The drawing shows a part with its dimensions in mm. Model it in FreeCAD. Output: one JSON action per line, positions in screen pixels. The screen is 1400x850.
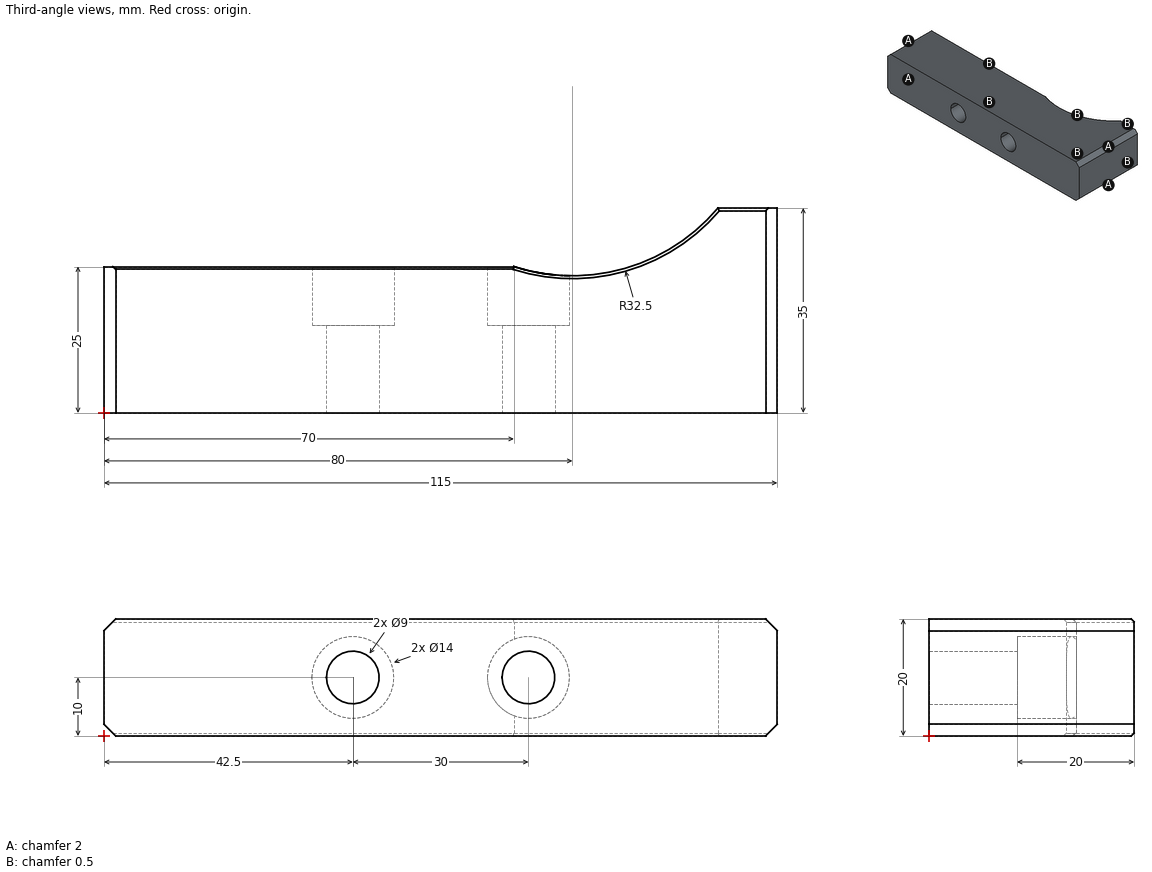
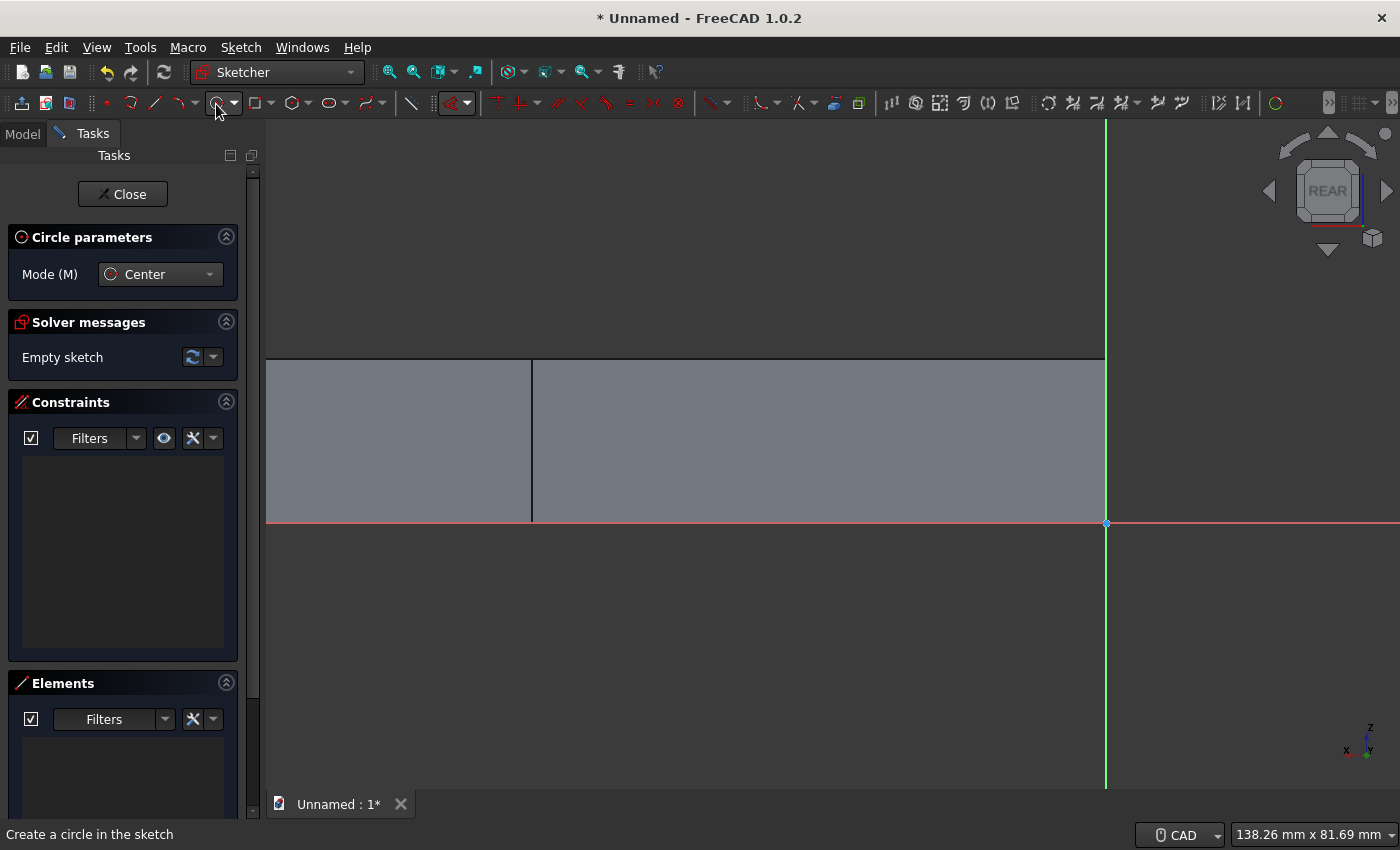
{"action": "left_click", "coordinate": [758, 441]}
{"action": "left_click", "coordinate": [798, 401]}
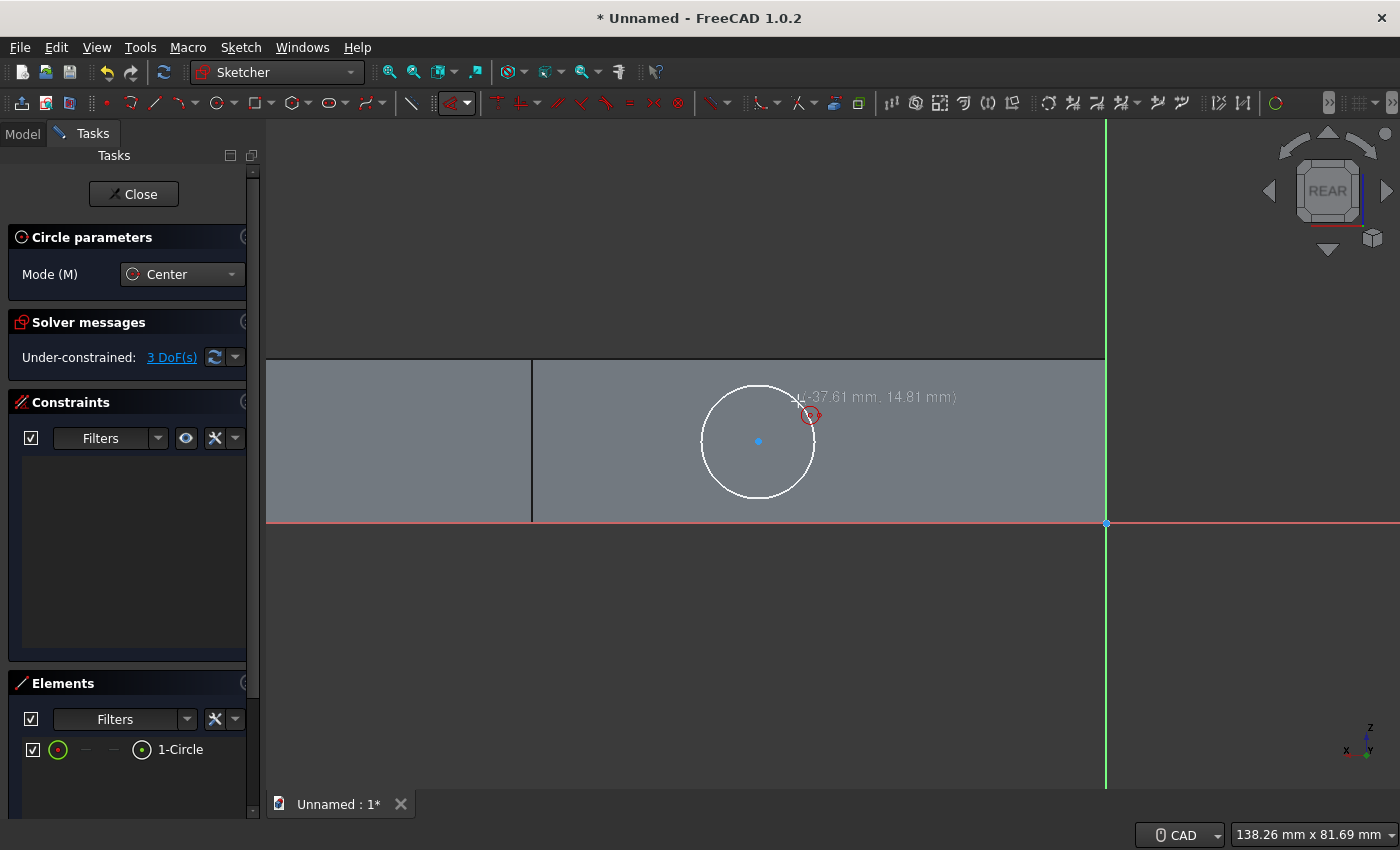
{"action": "left_click", "coordinate": [512, 441]}
{"action": "left_click", "coordinate": [552, 401]}
{"action": "key", "text": "Escape"}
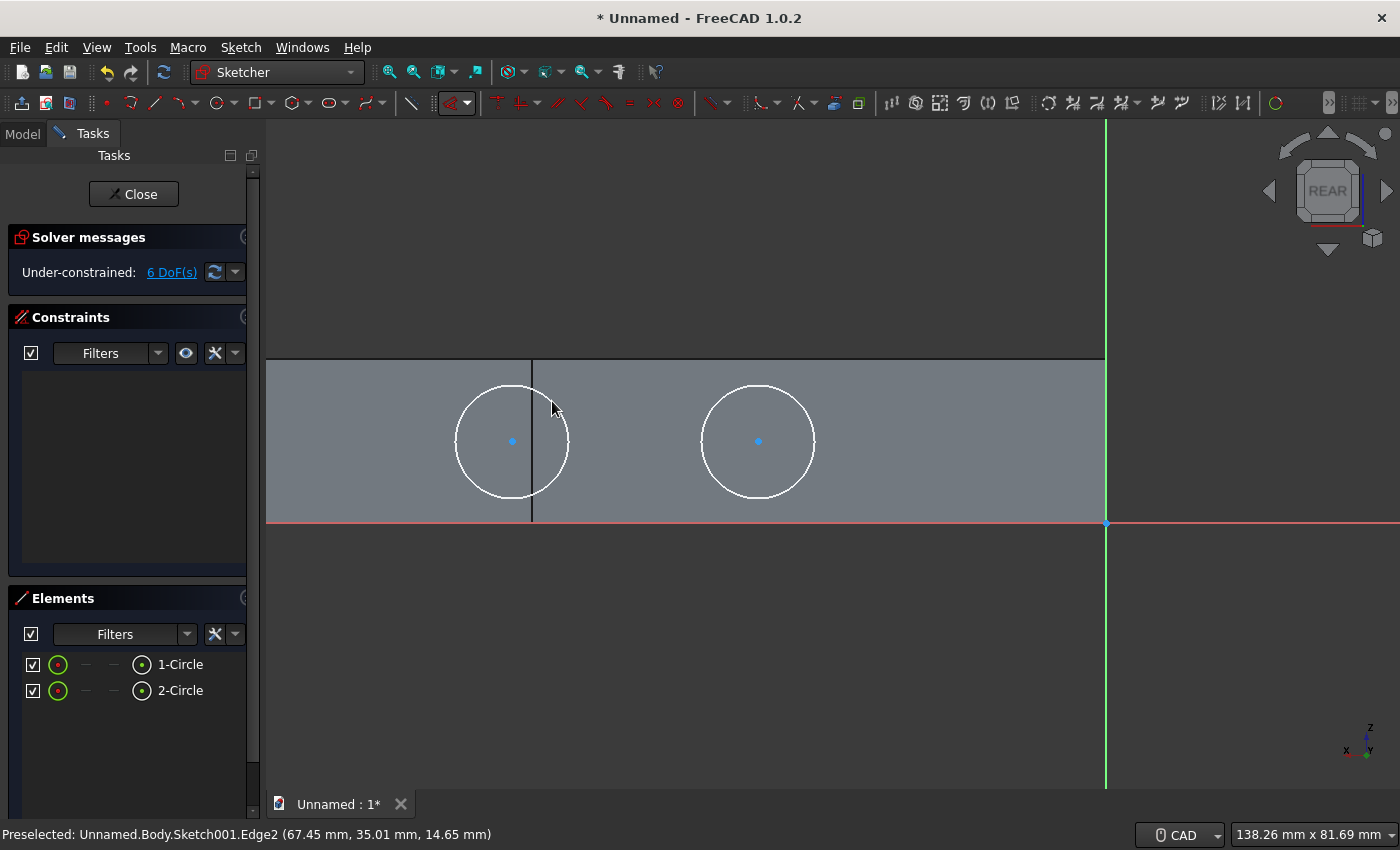
{"action": "left_click", "coordinate": [798, 402]}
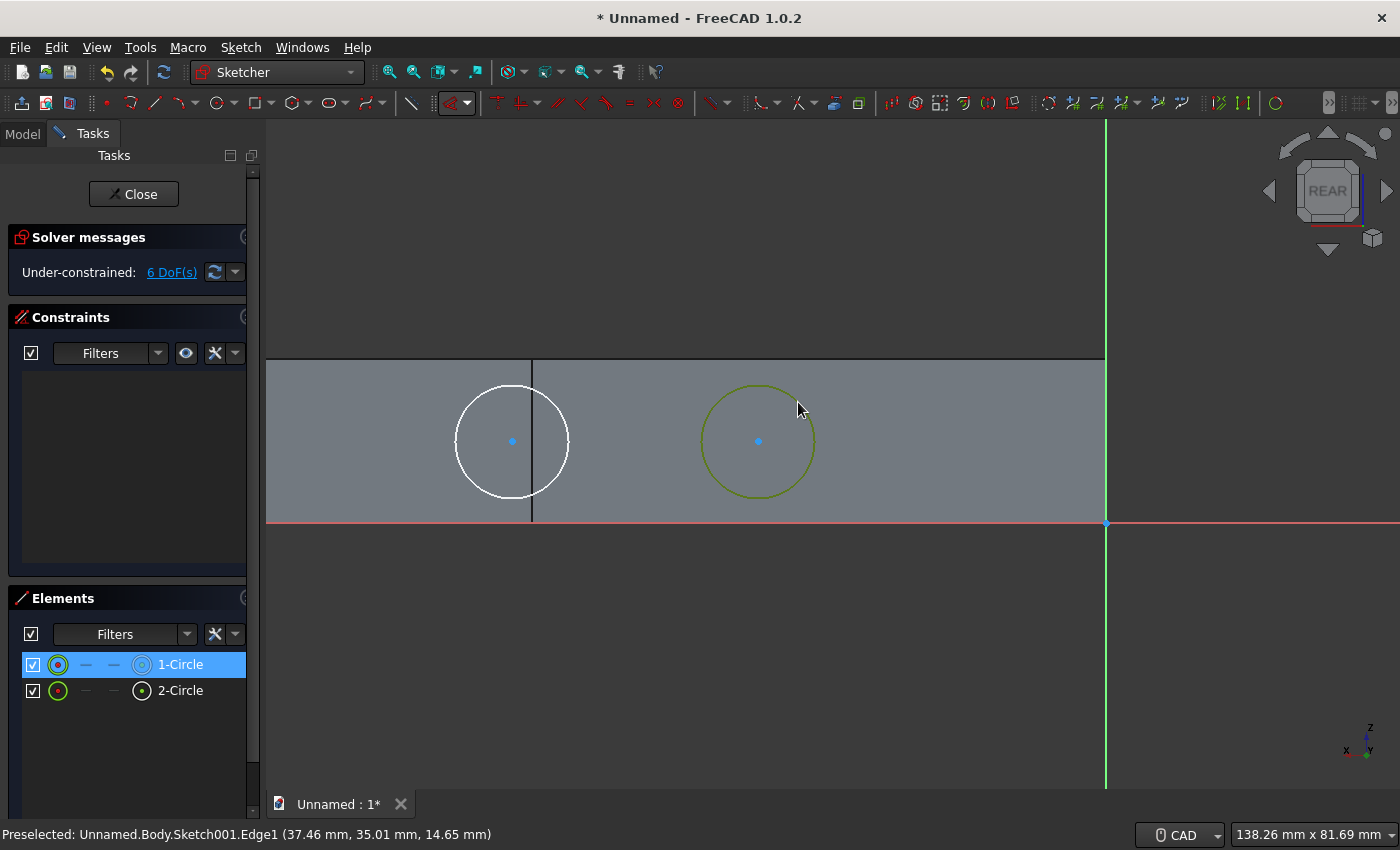
{"action": "left_click", "coordinate": [552, 402]}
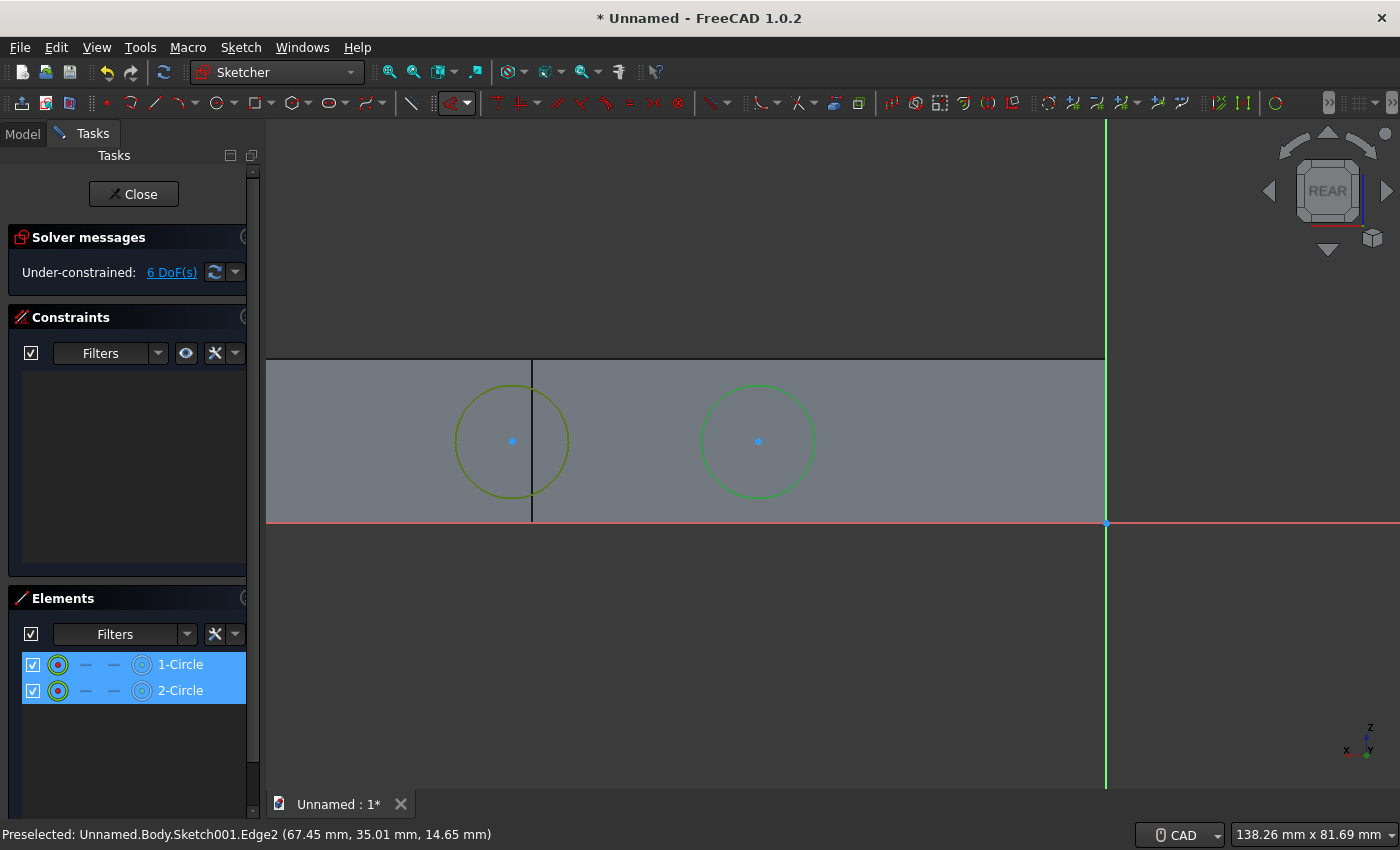
{"action": "left_click", "coordinate": [630, 104]}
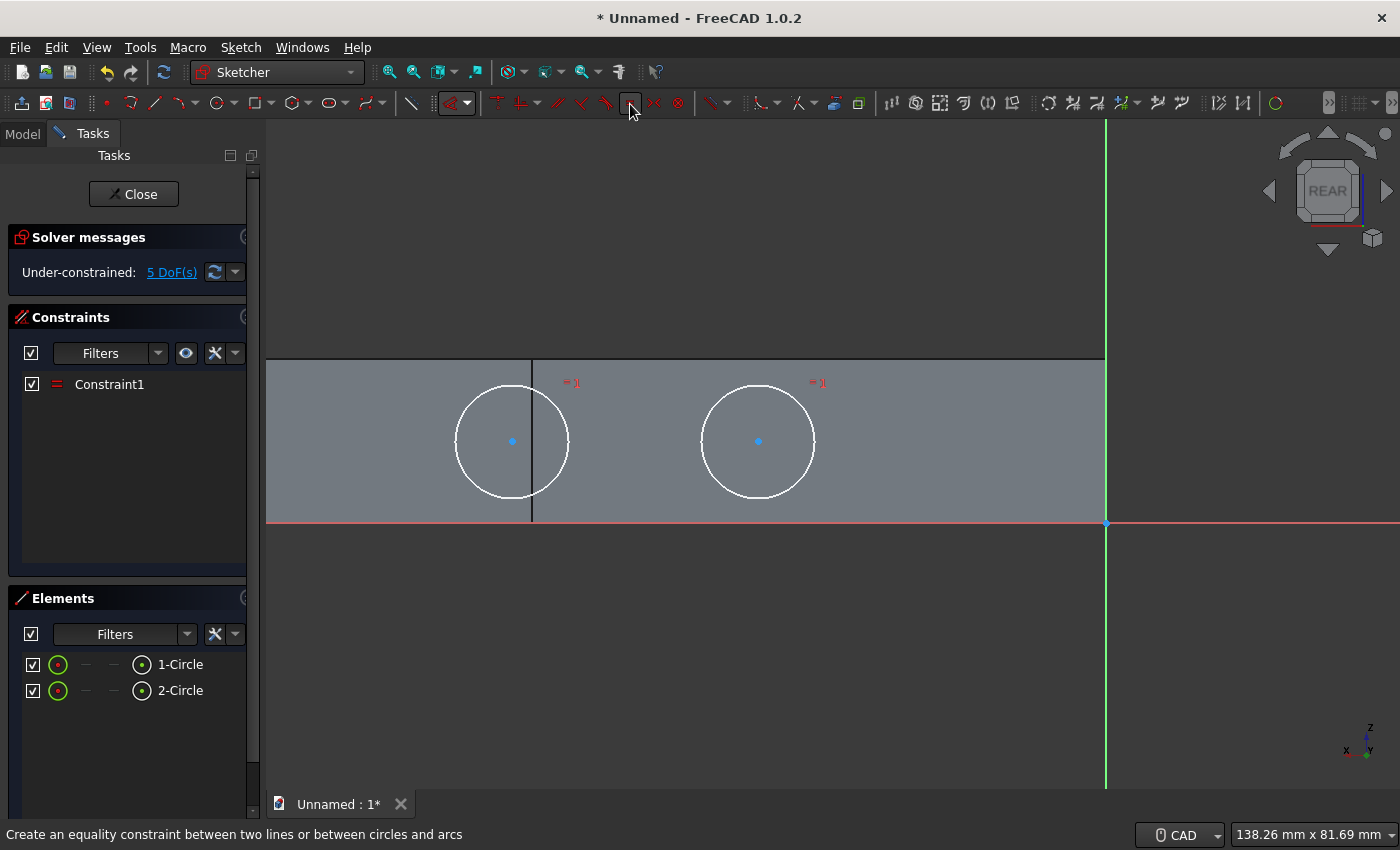
{"action": "left_click", "coordinate": [758, 442]}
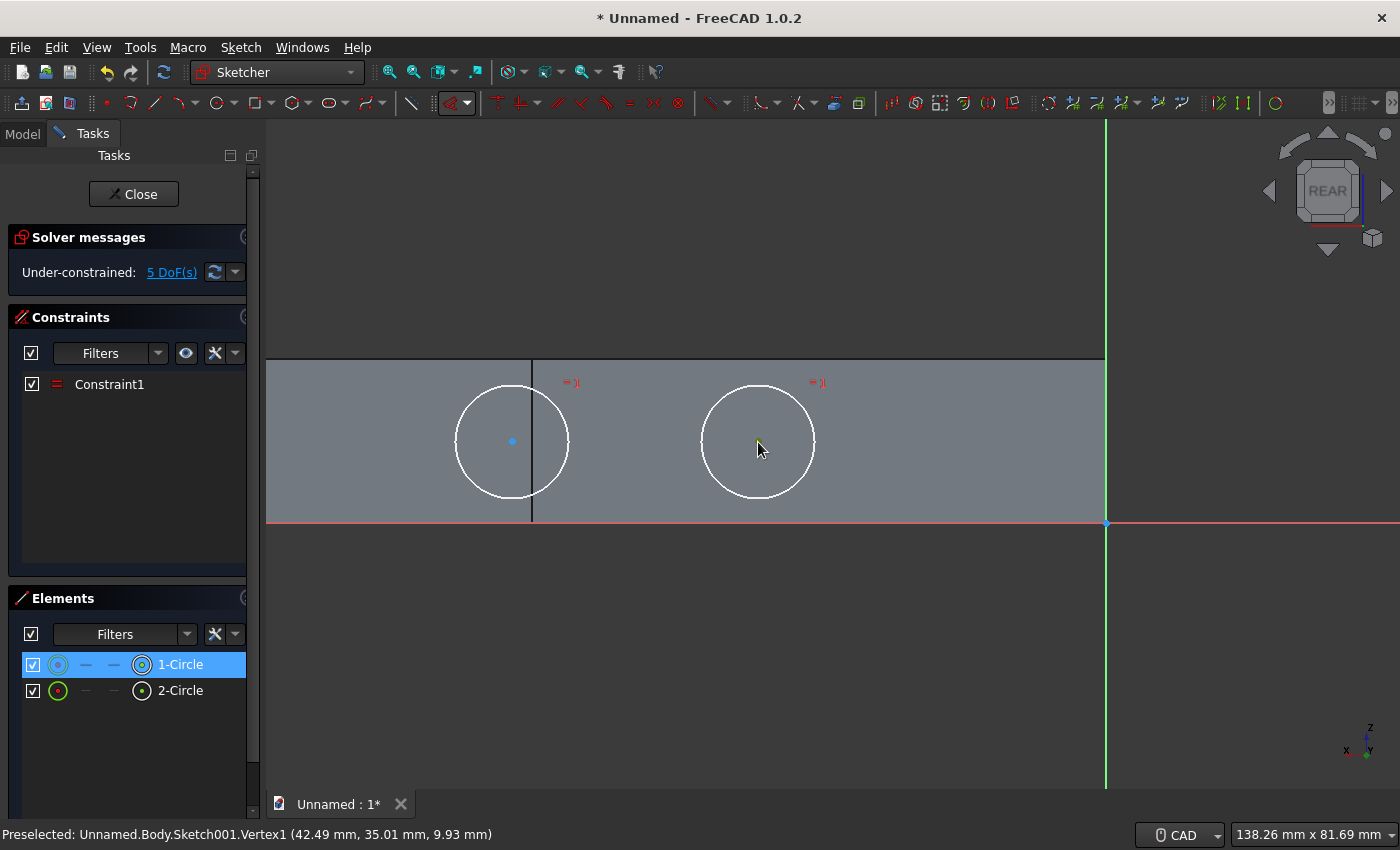
{"action": "left_click", "coordinate": [512, 442]}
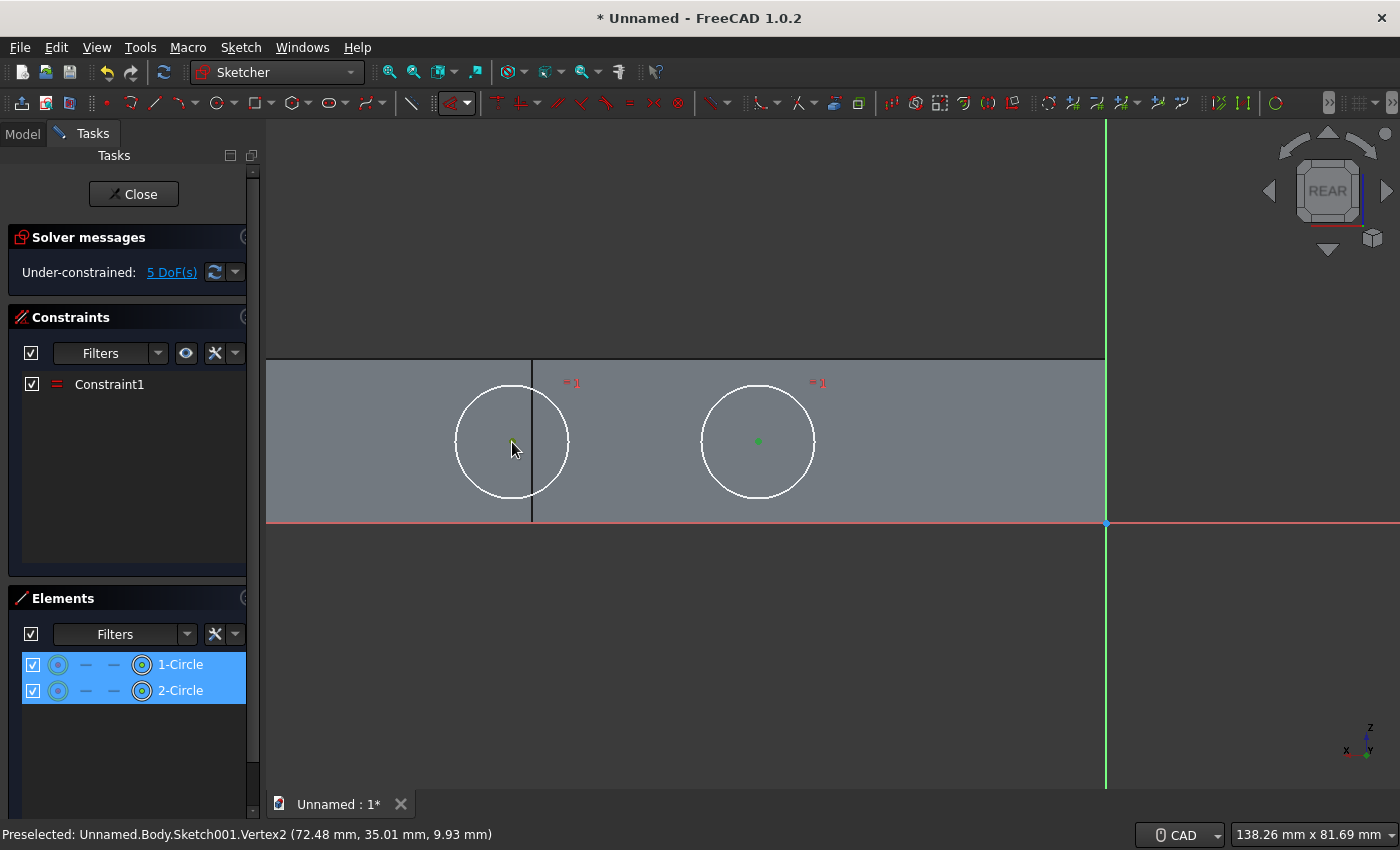
{"action": "left_click", "coordinate": [540, 104]}